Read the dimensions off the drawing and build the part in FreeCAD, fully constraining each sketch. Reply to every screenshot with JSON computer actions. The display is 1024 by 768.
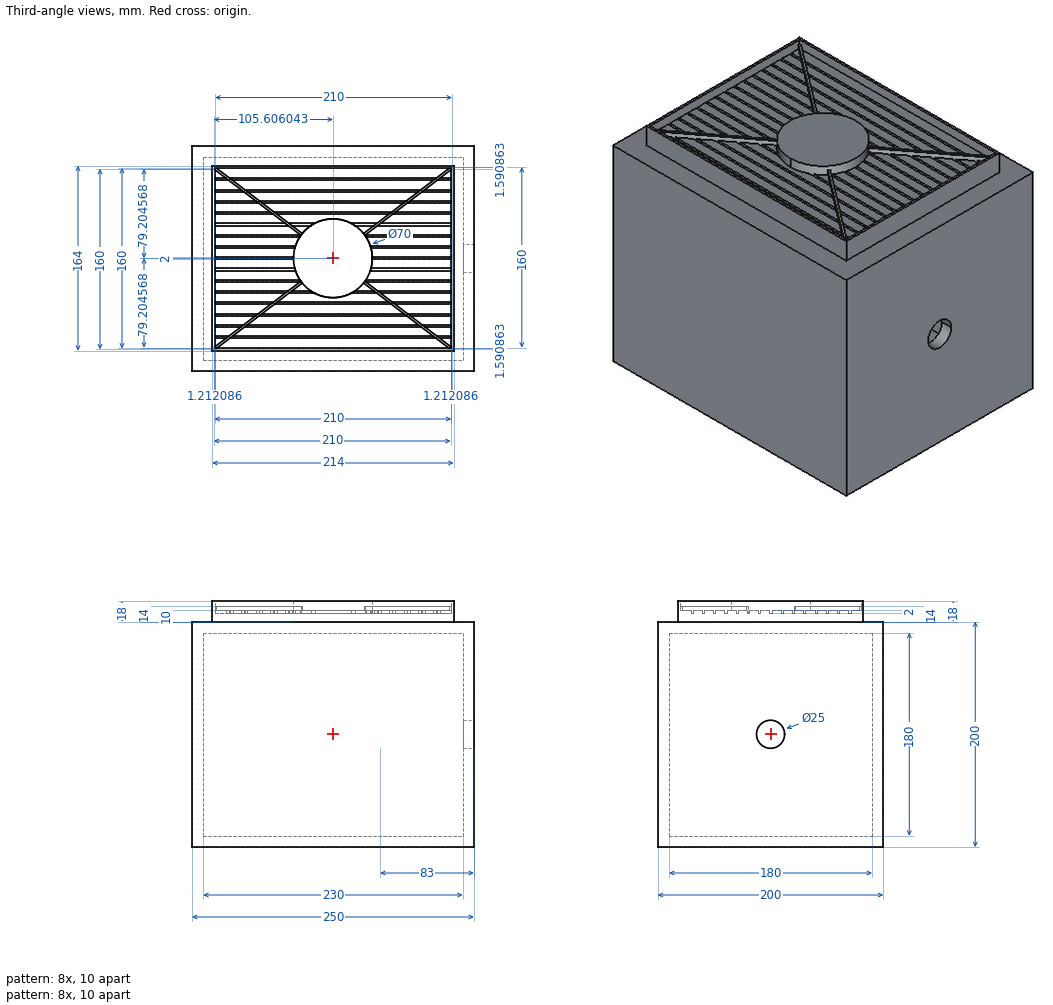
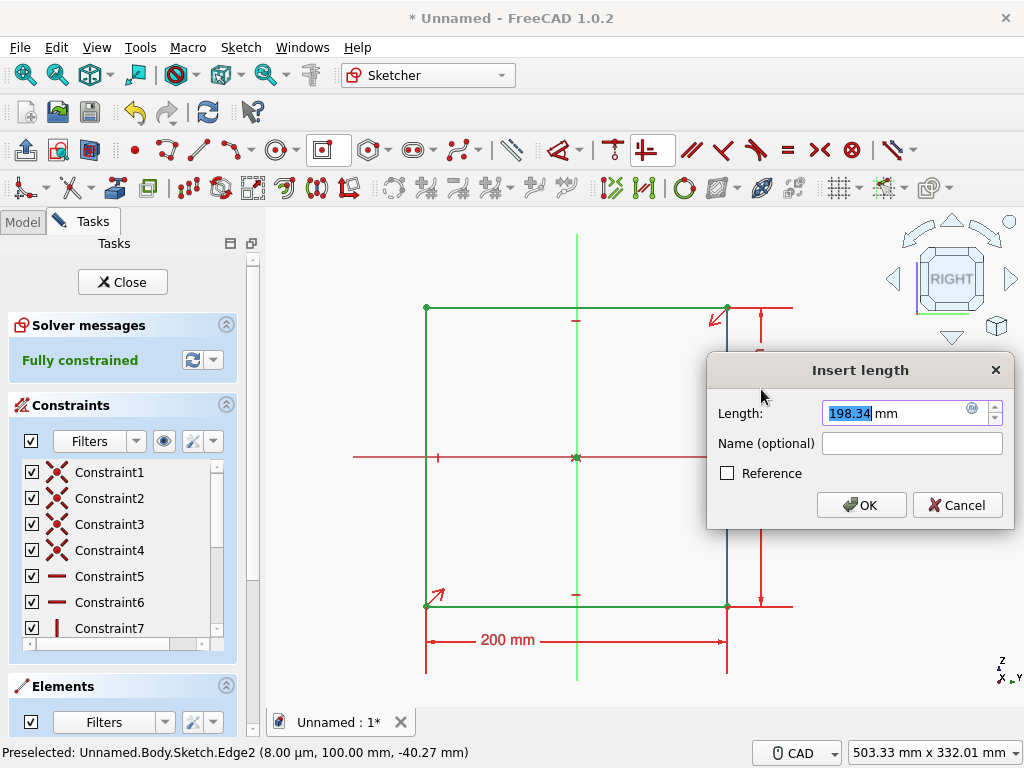
{"action": "type", "text": "200"}
{"action": "key", "text": "Return"}
{"action": "key", "text": "Escape"}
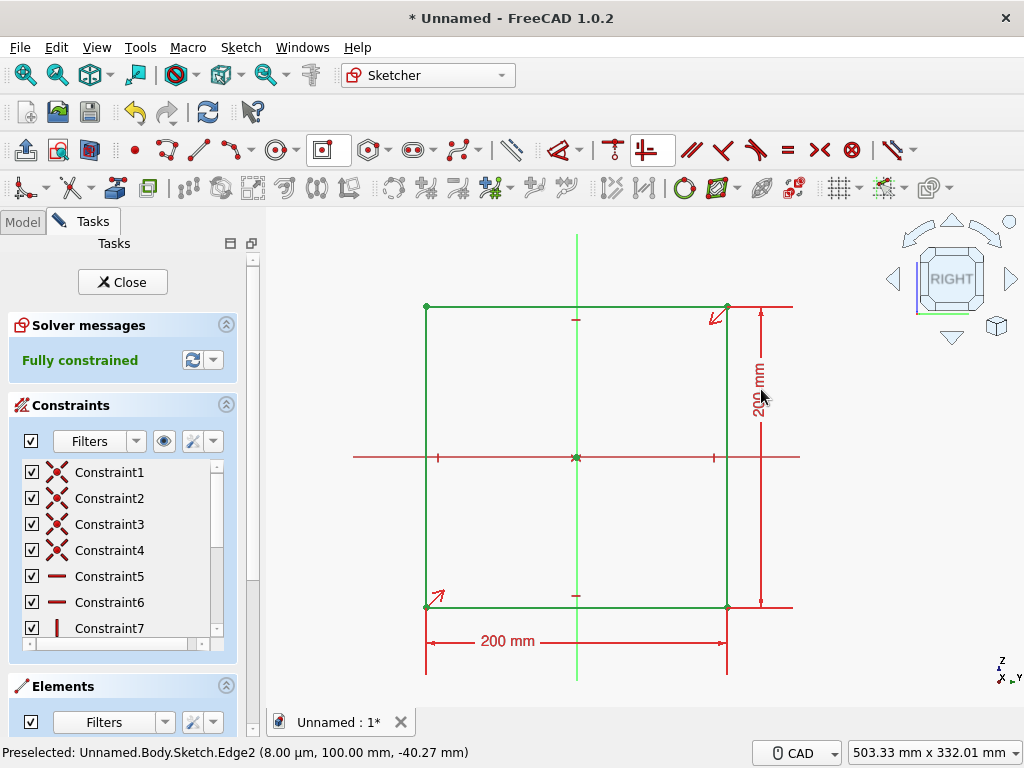
{"action": "left_click", "coordinate": [123, 282]}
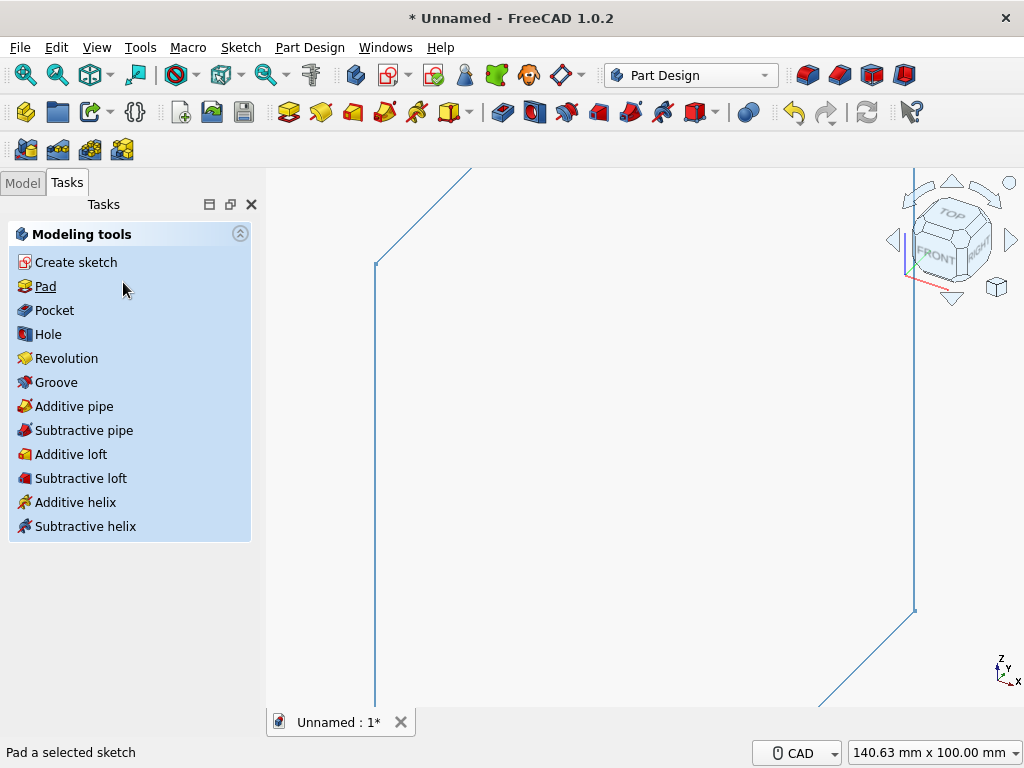
{"action": "left_click", "coordinate": [290, 112]}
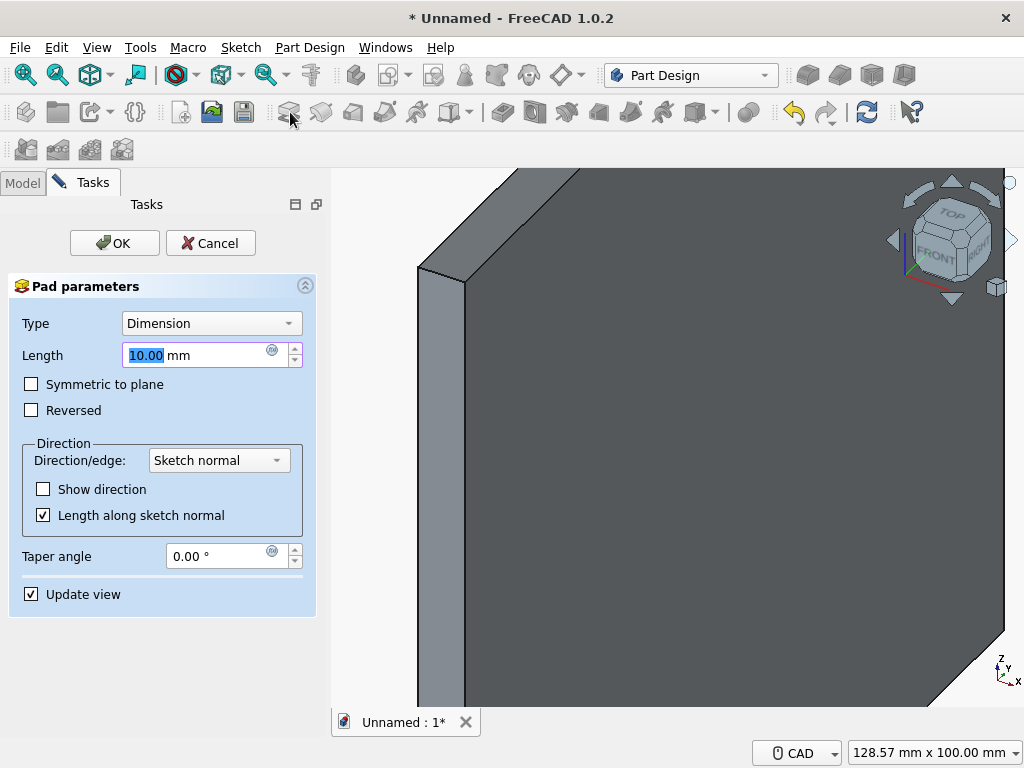
{"action": "type", "text": "250"}
{"action": "key", "text": "Tab"}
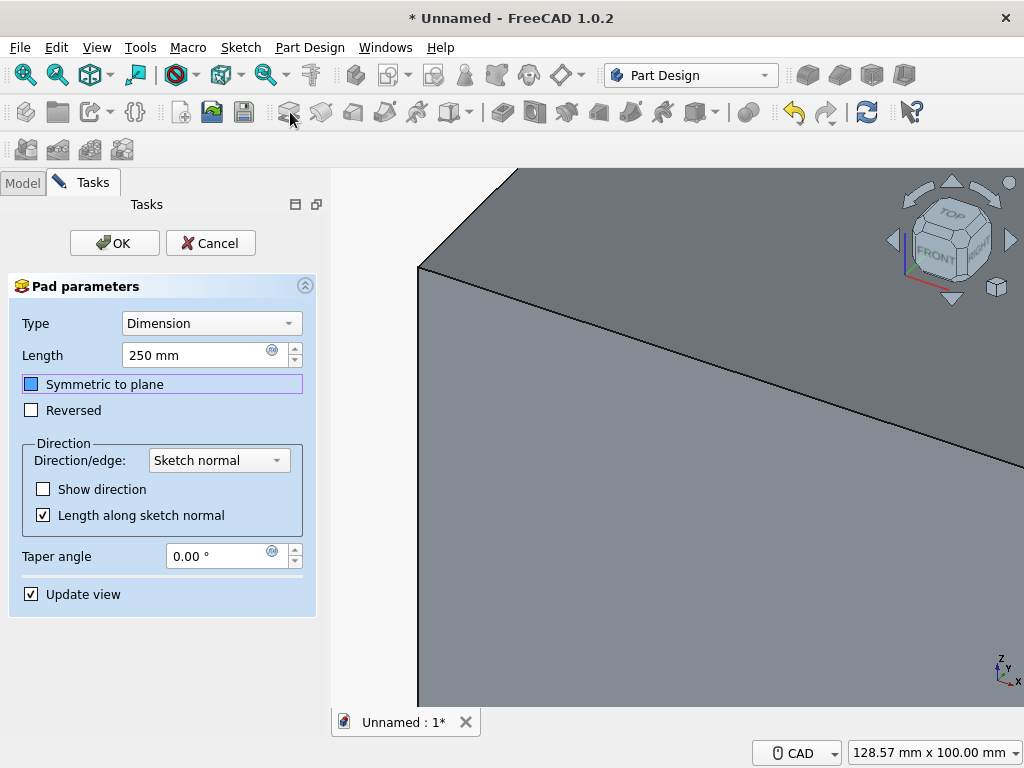
{"action": "left_click", "coordinate": [30, 384]}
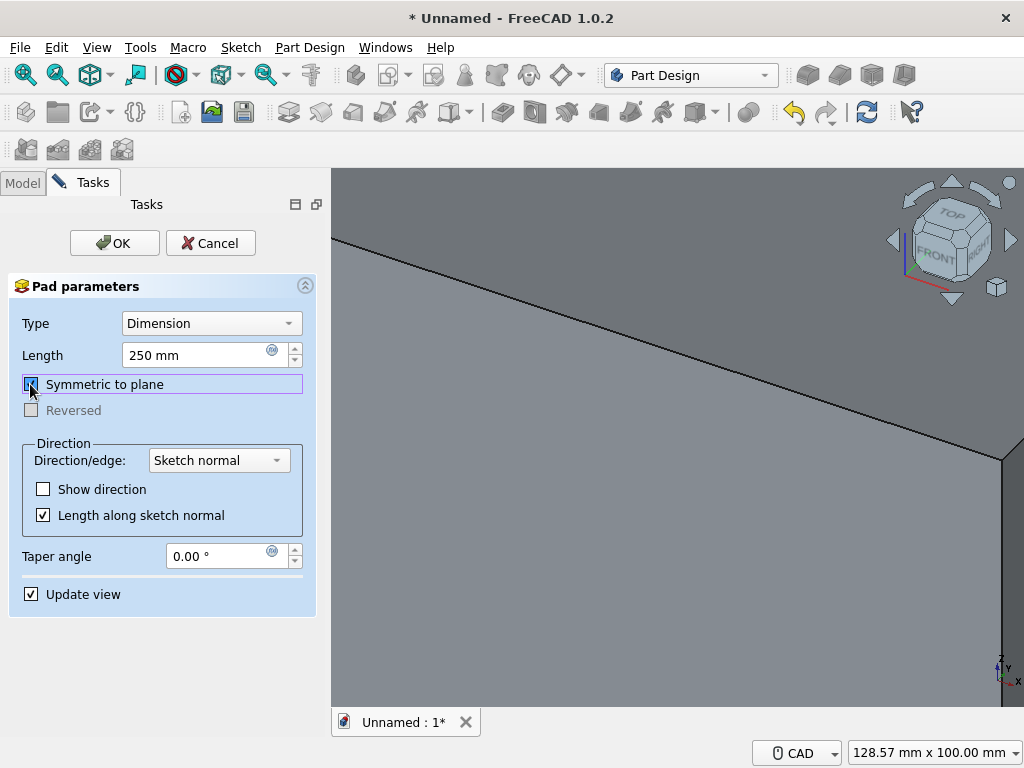
{"action": "left_click", "coordinate": [115, 243]}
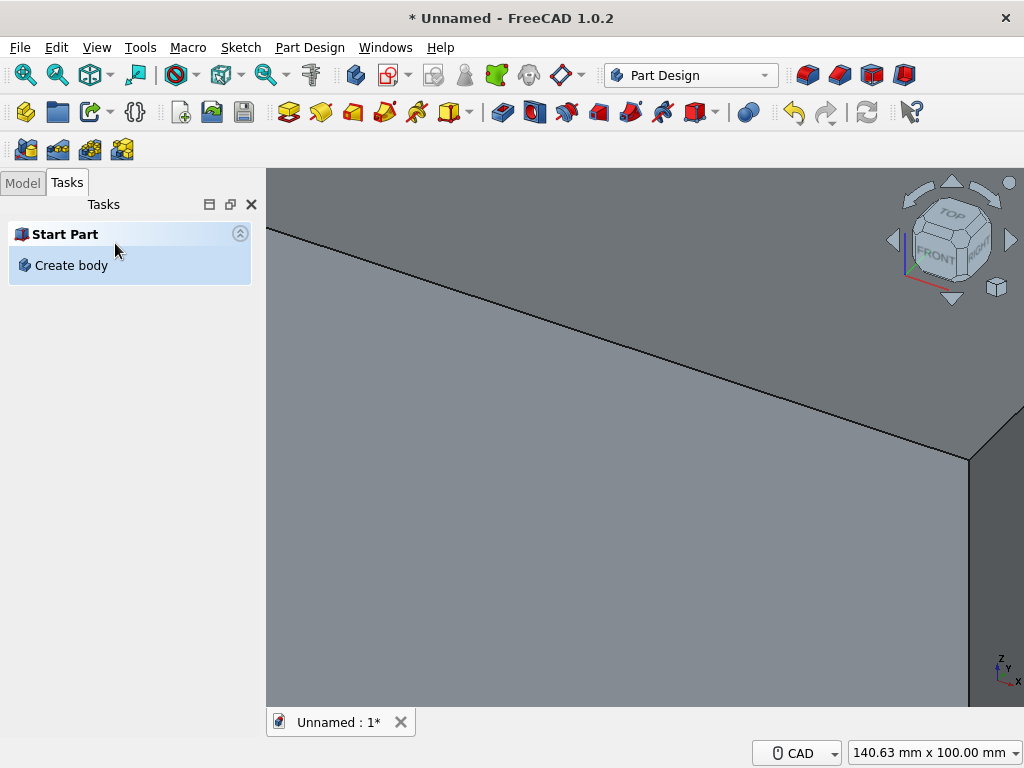
{"action": "left_click", "coordinate": [26, 76]}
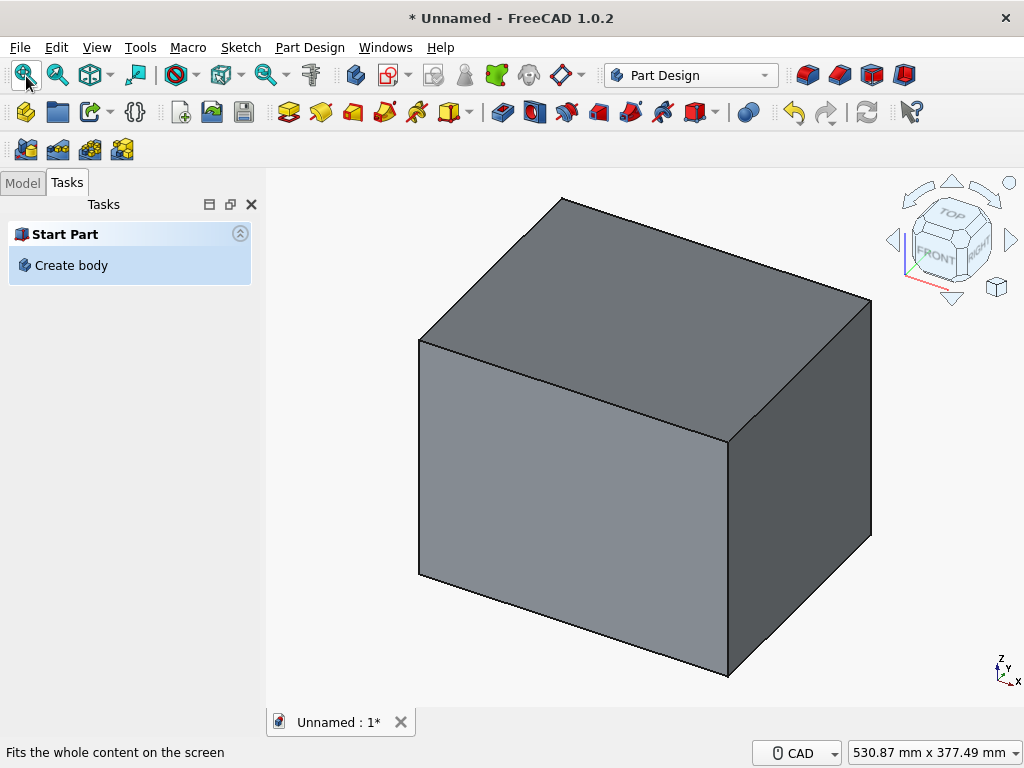
{"action": "left_click", "coordinate": [645, 320]}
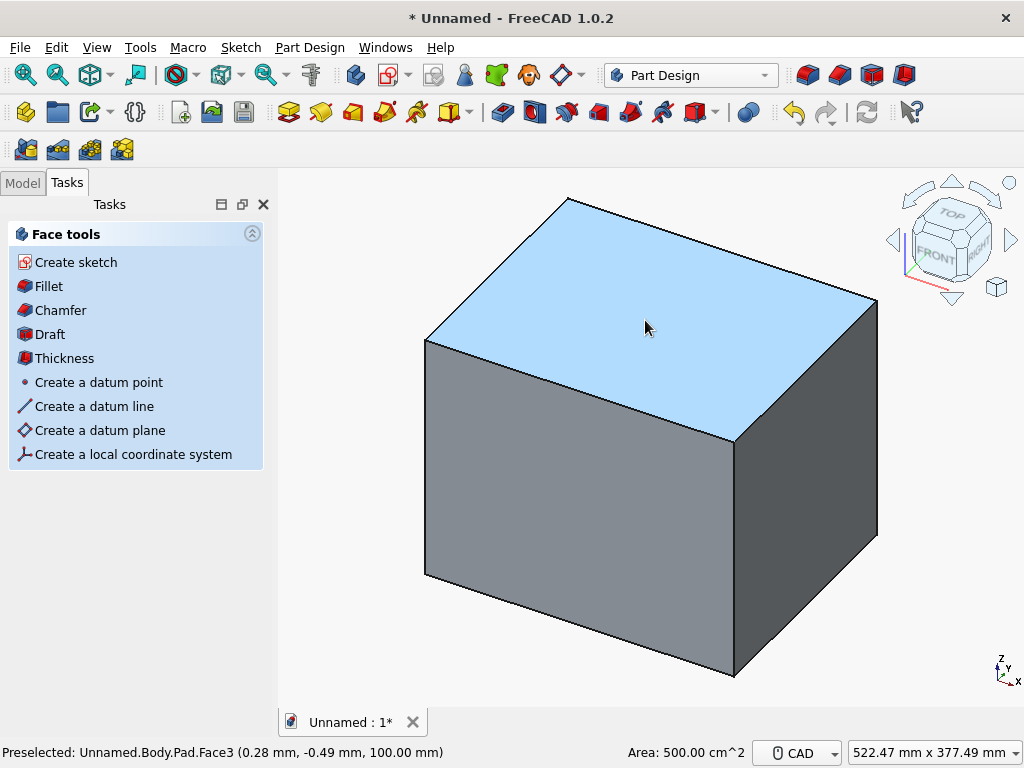
{"action": "left_click", "coordinate": [388, 76]}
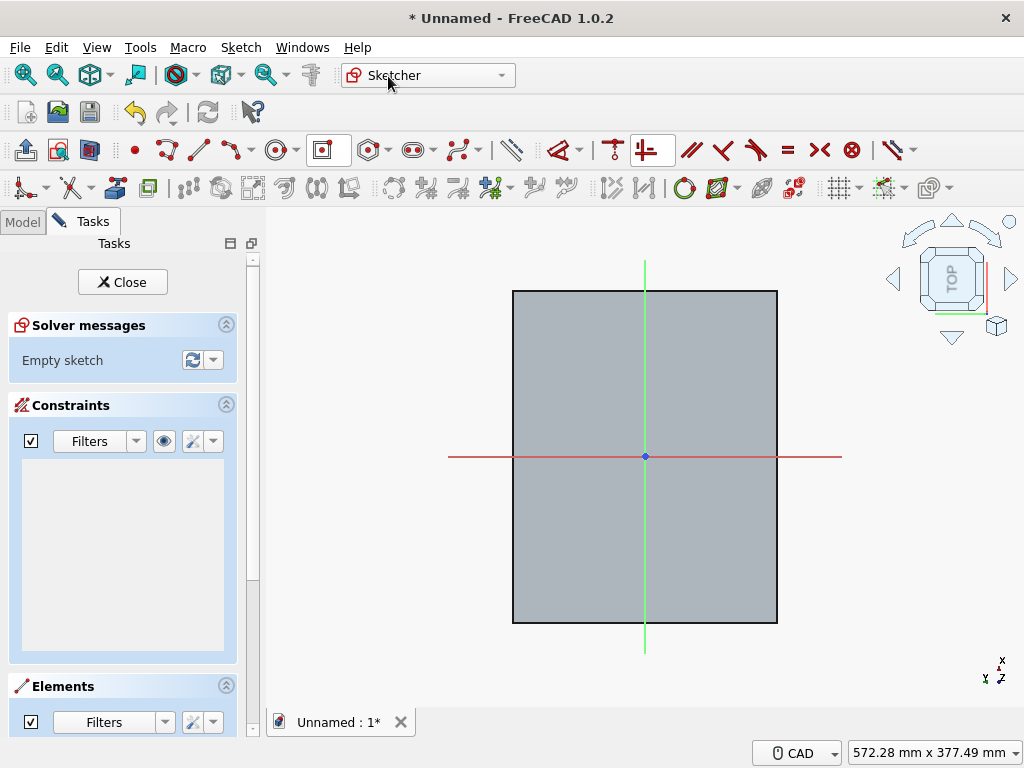
{"action": "left_click", "coordinate": [322, 150]}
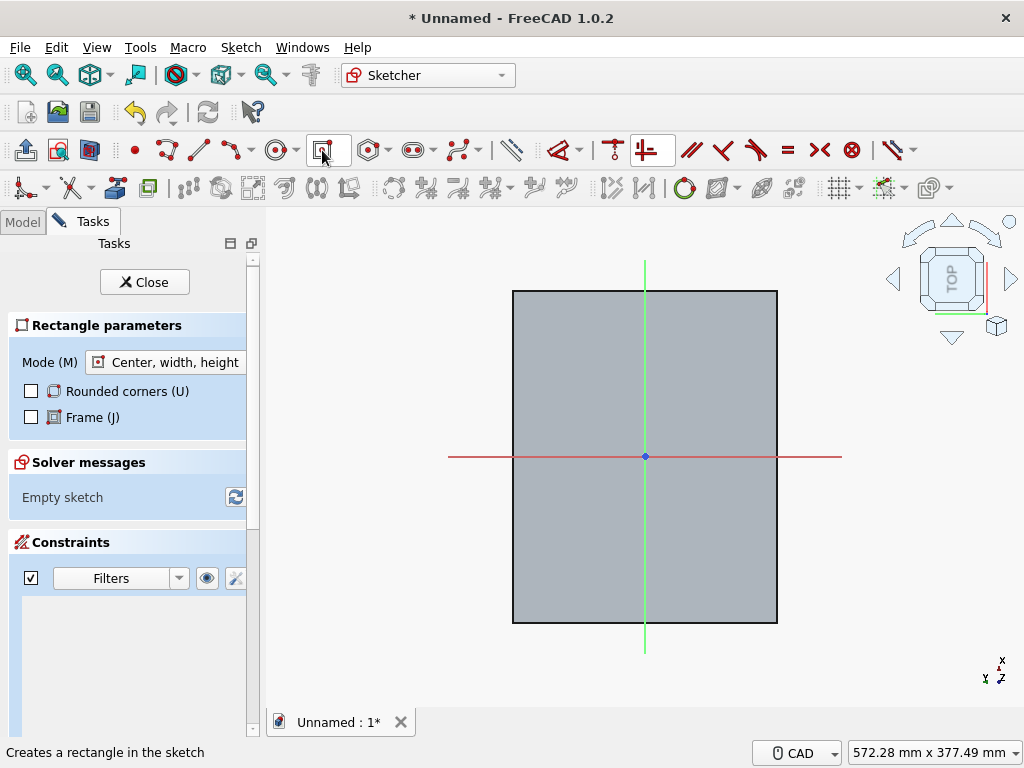
{"action": "left_click", "coordinate": [645, 457]}
{"action": "left_click", "coordinate": [751, 318]}
{"action": "key", "text": "Escape"}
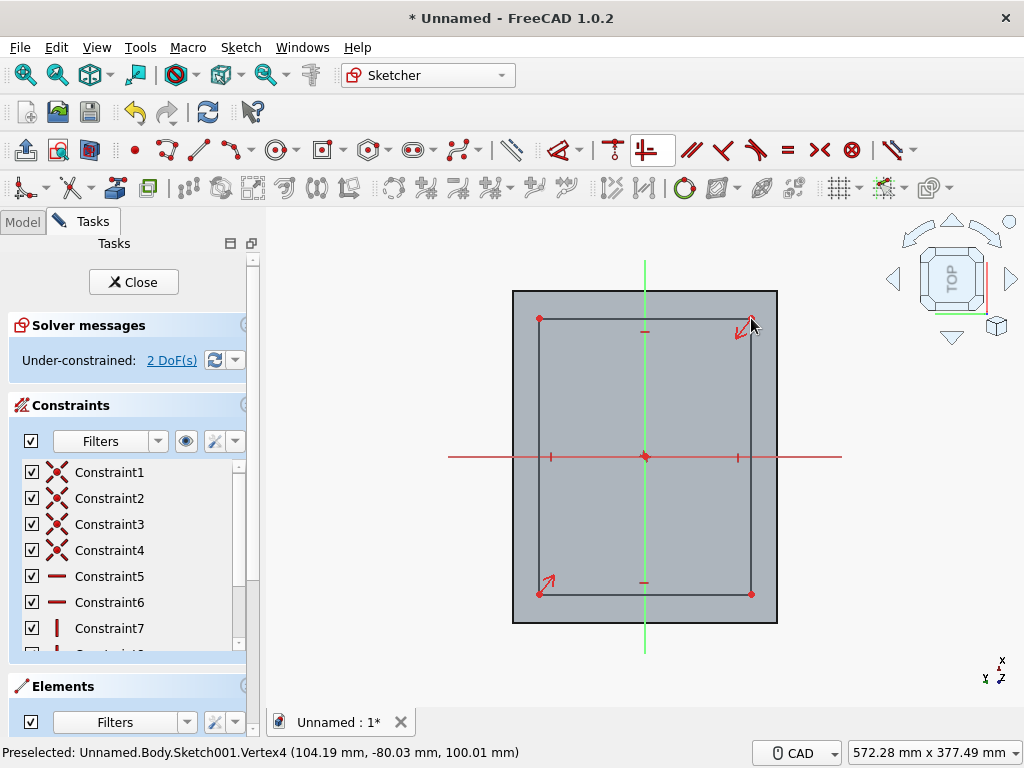
{"action": "left_click", "coordinate": [558, 150]}